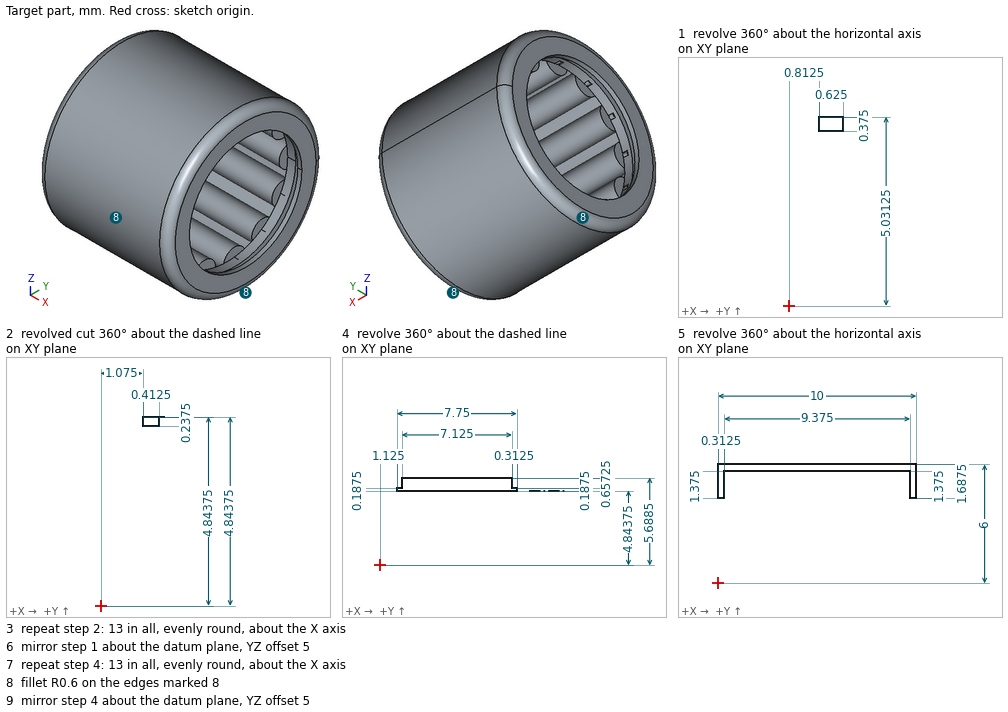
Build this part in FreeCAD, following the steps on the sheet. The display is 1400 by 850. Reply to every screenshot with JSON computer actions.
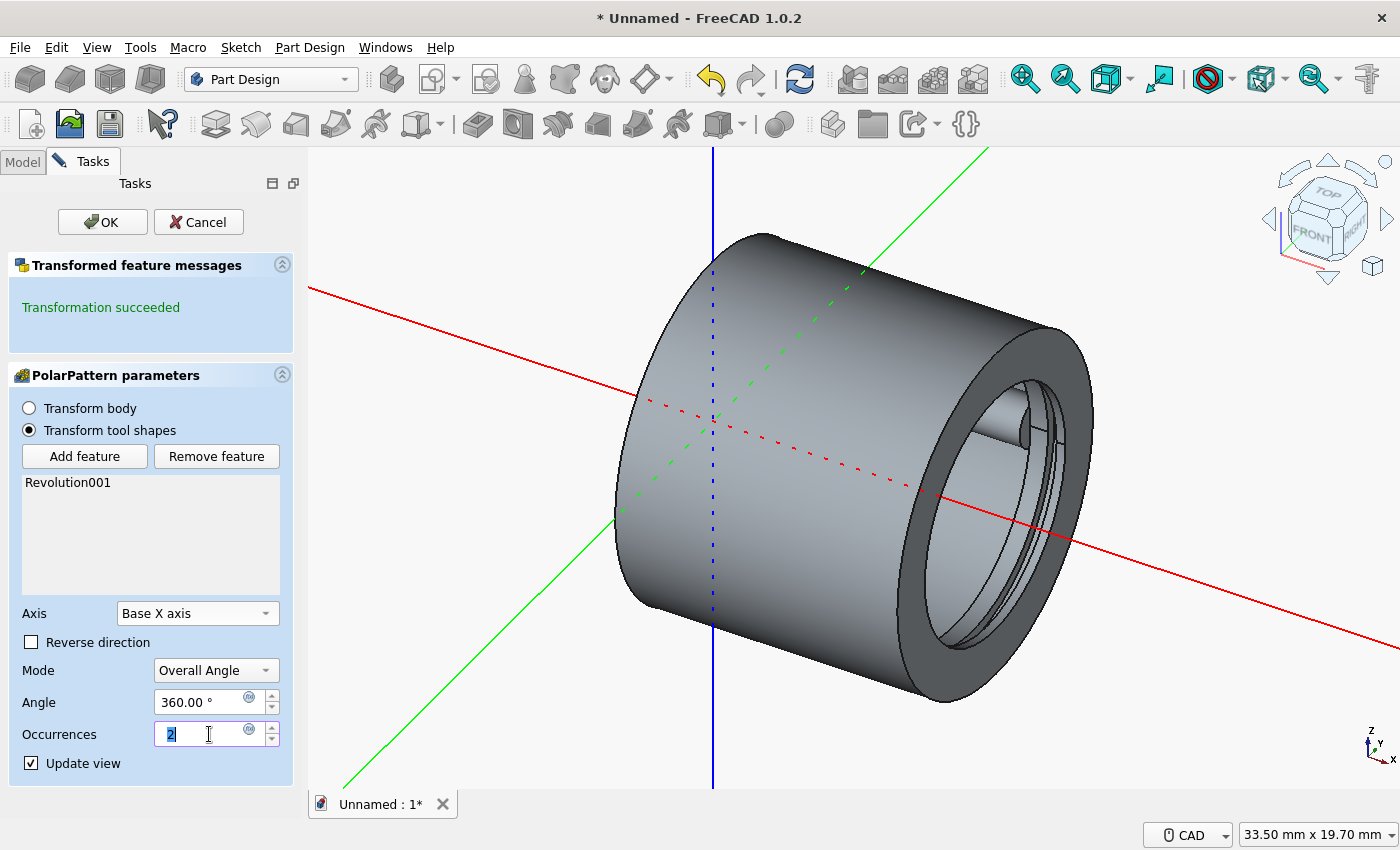
{"action": "type", "text": "13"}
{"action": "key", "text": "Tab"}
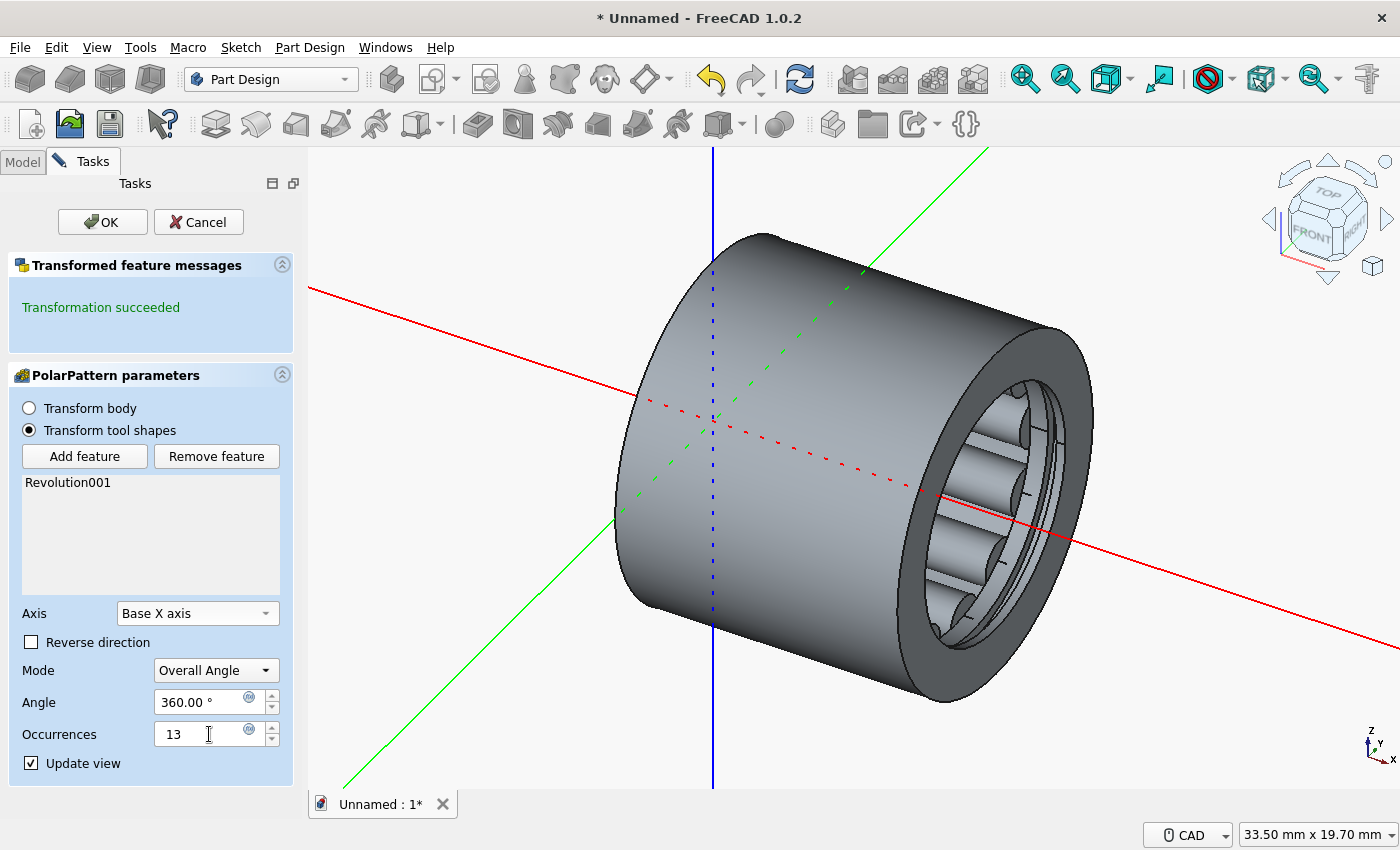
{"action": "left_click", "coordinate": [103, 222]}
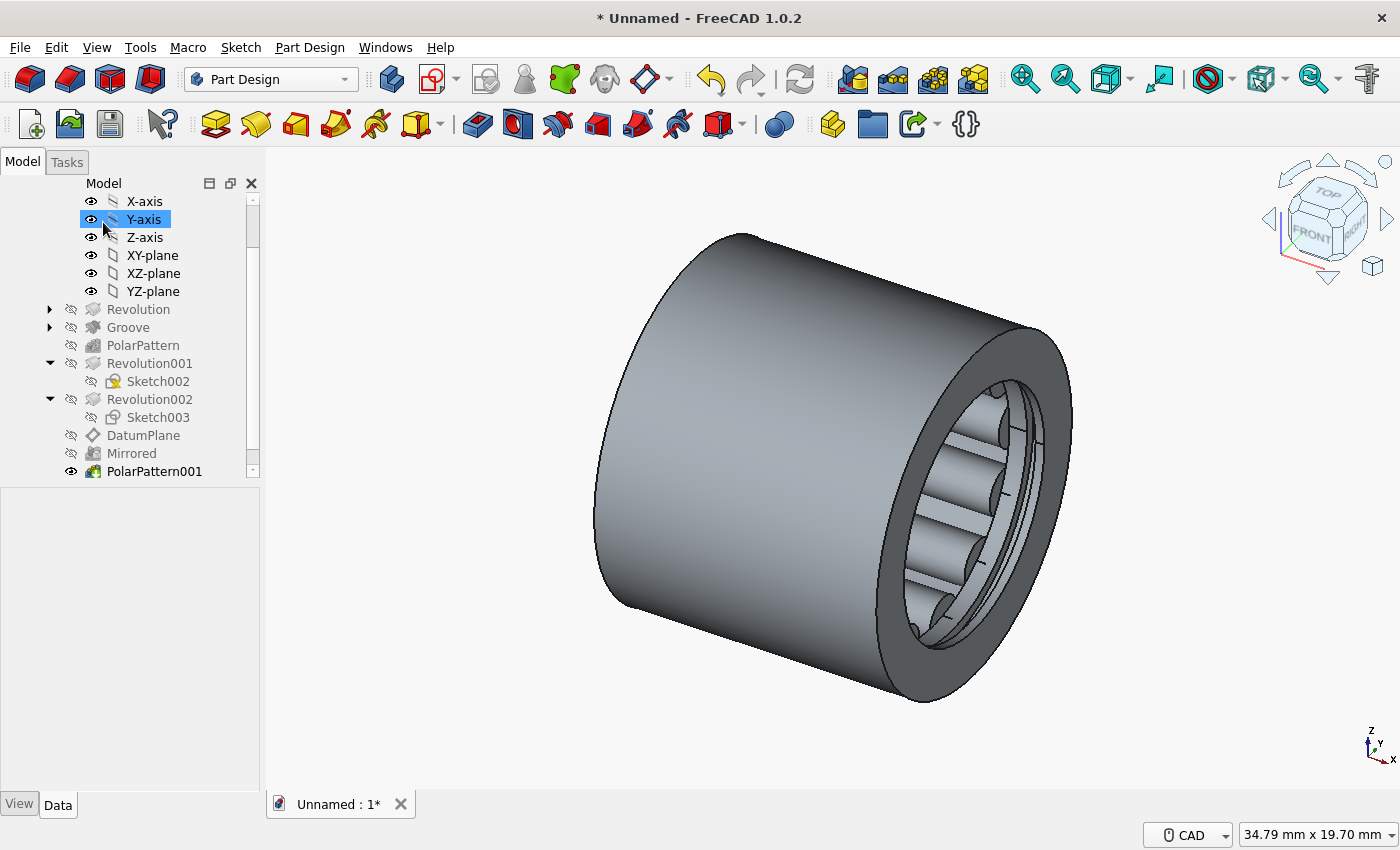
{"action": "left_click", "coordinate": [876, 611]}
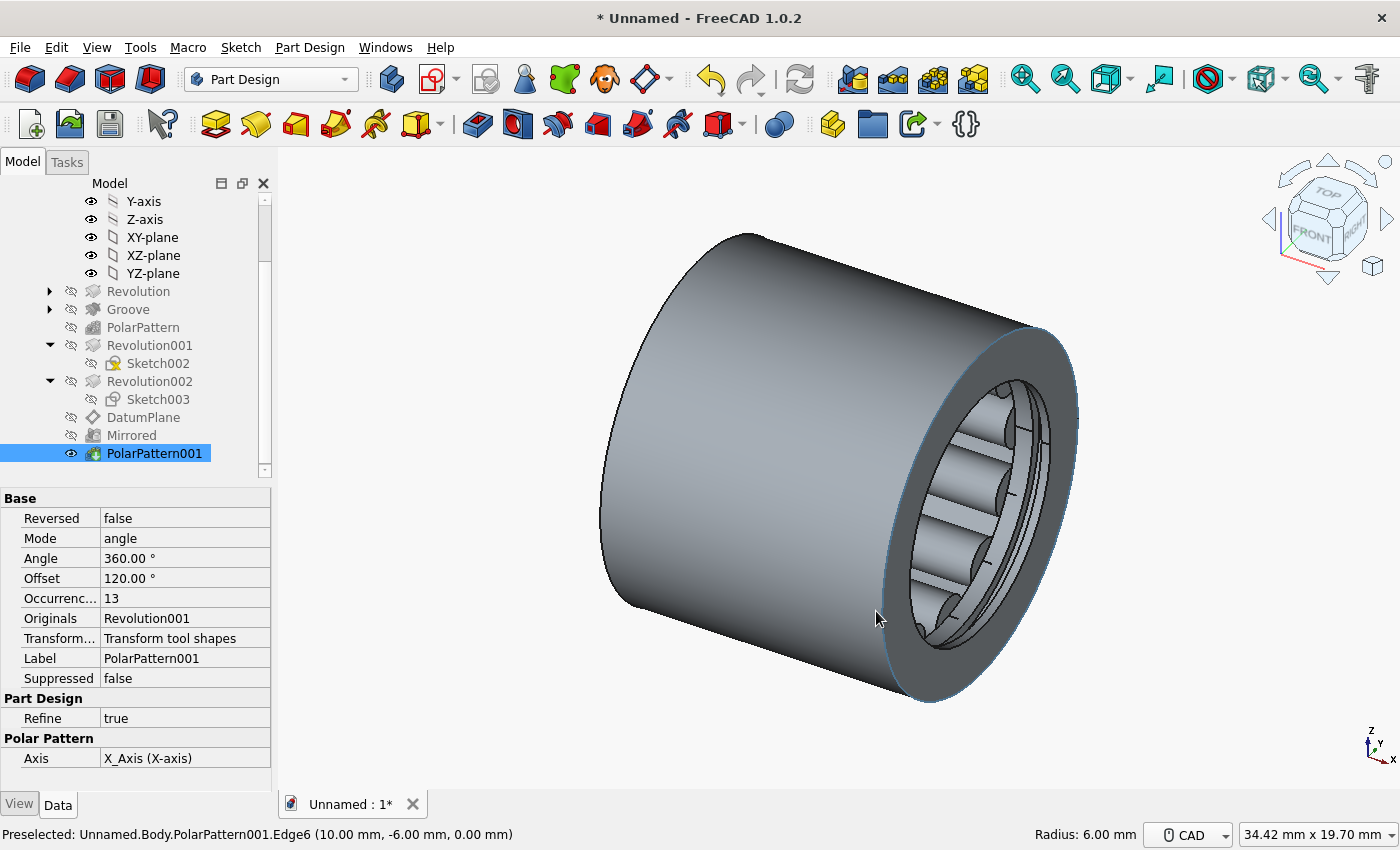
{"action": "key", "text": "0"}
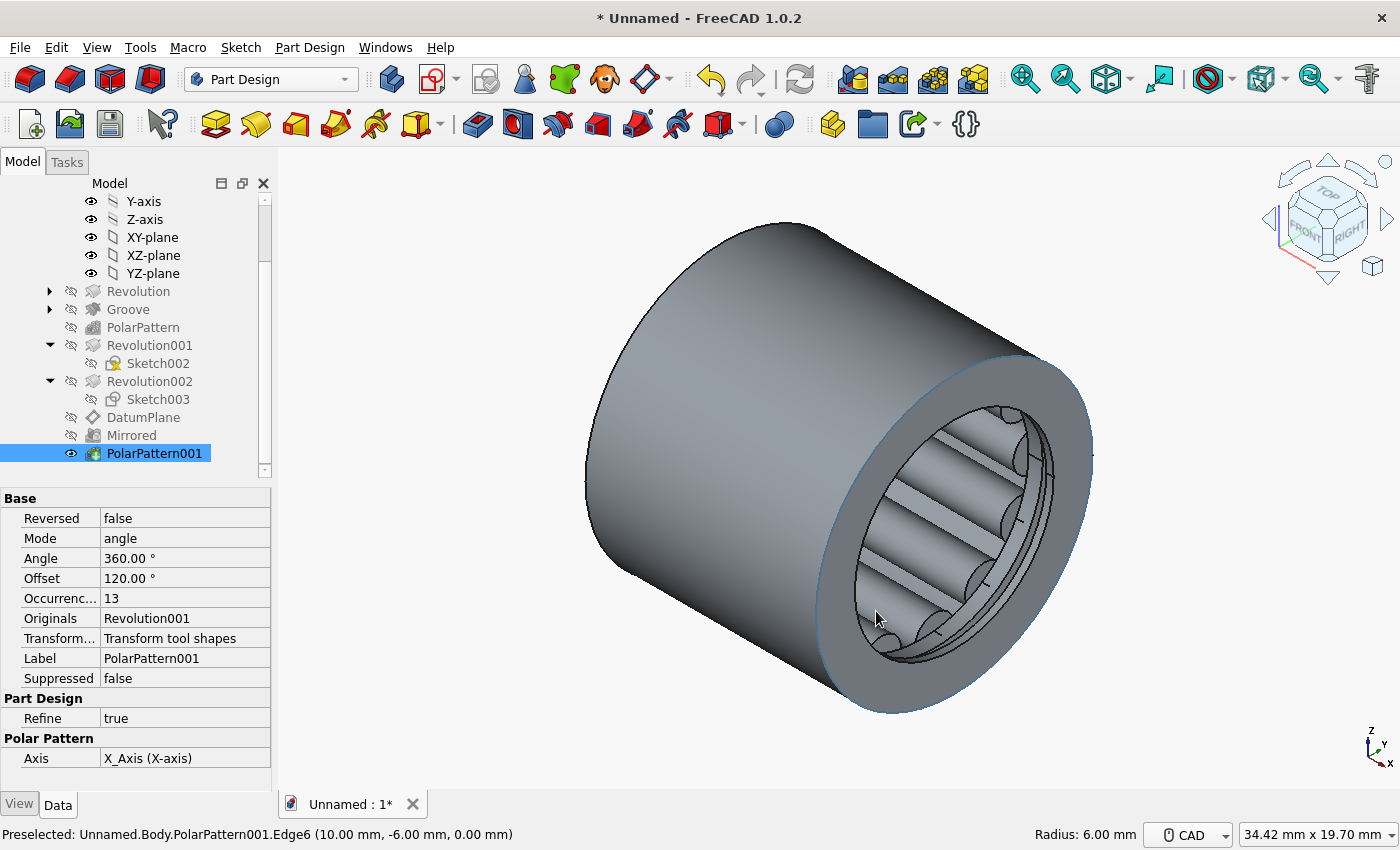
{"action": "key", "text": "2"}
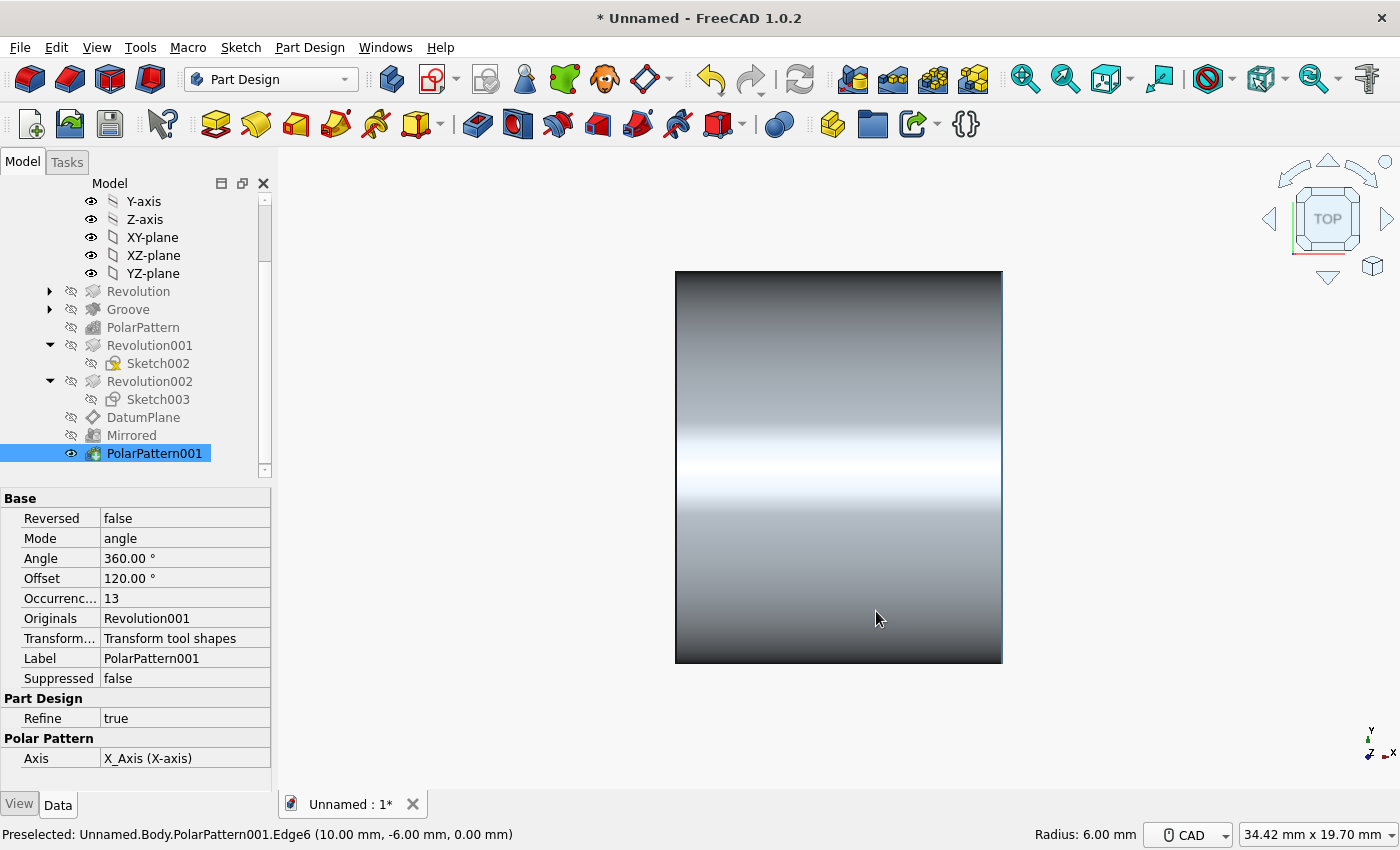
{"action": "left_click", "coordinate": [676, 625], "text": "ctrl"}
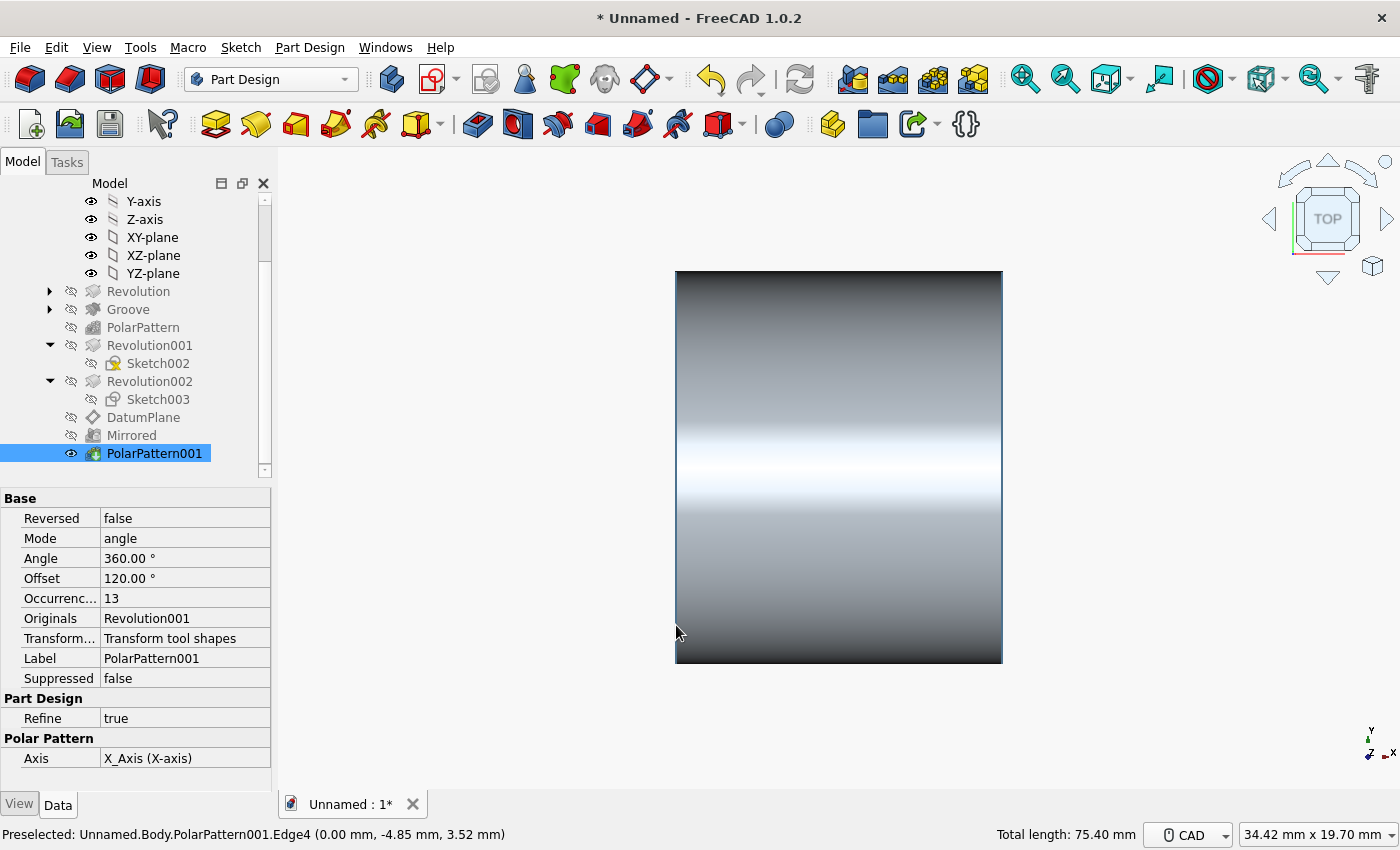
{"action": "left_click", "coordinate": [30, 80]}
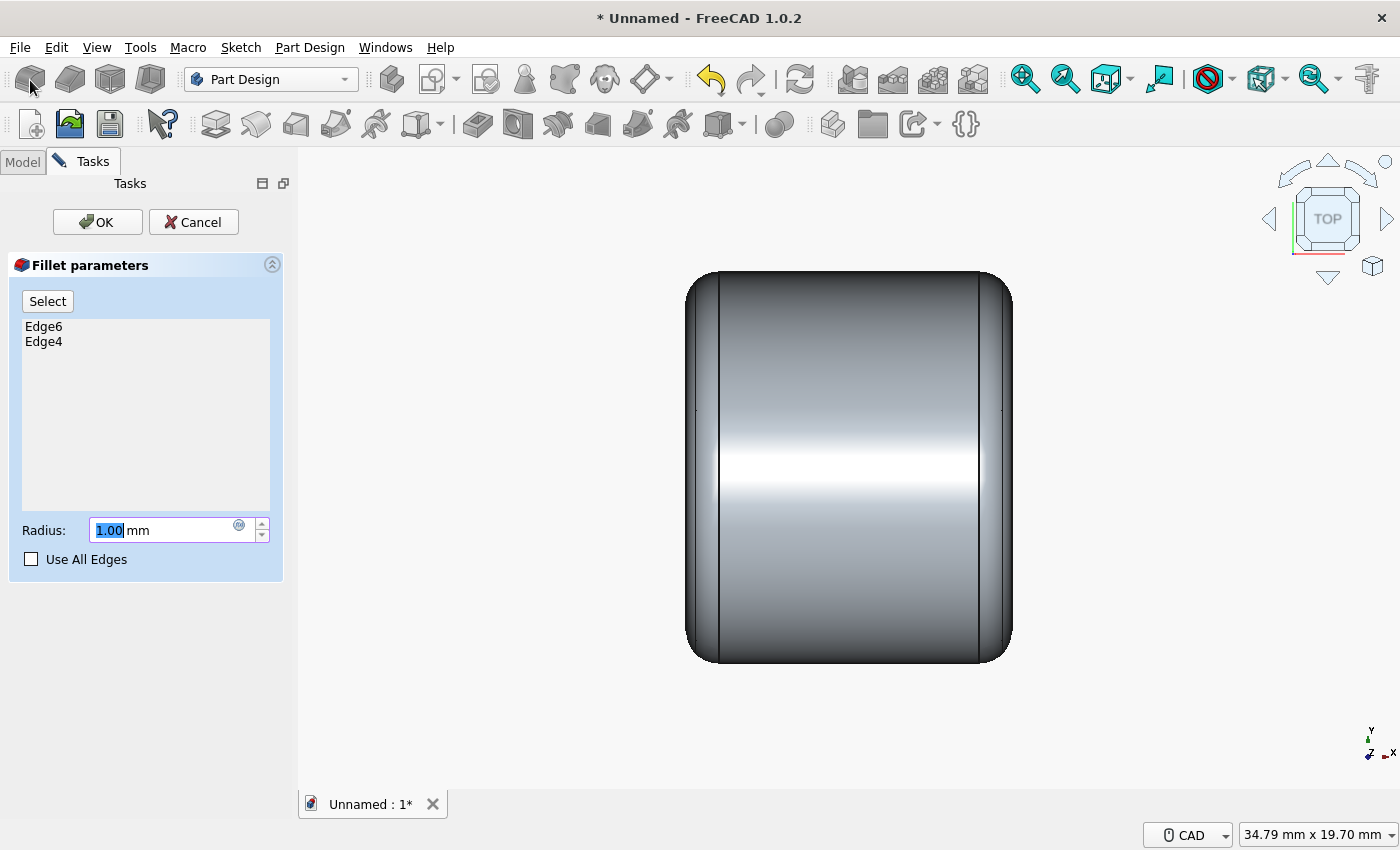
{"action": "type", "text": "0.6"}
{"action": "key", "text": "Tab"}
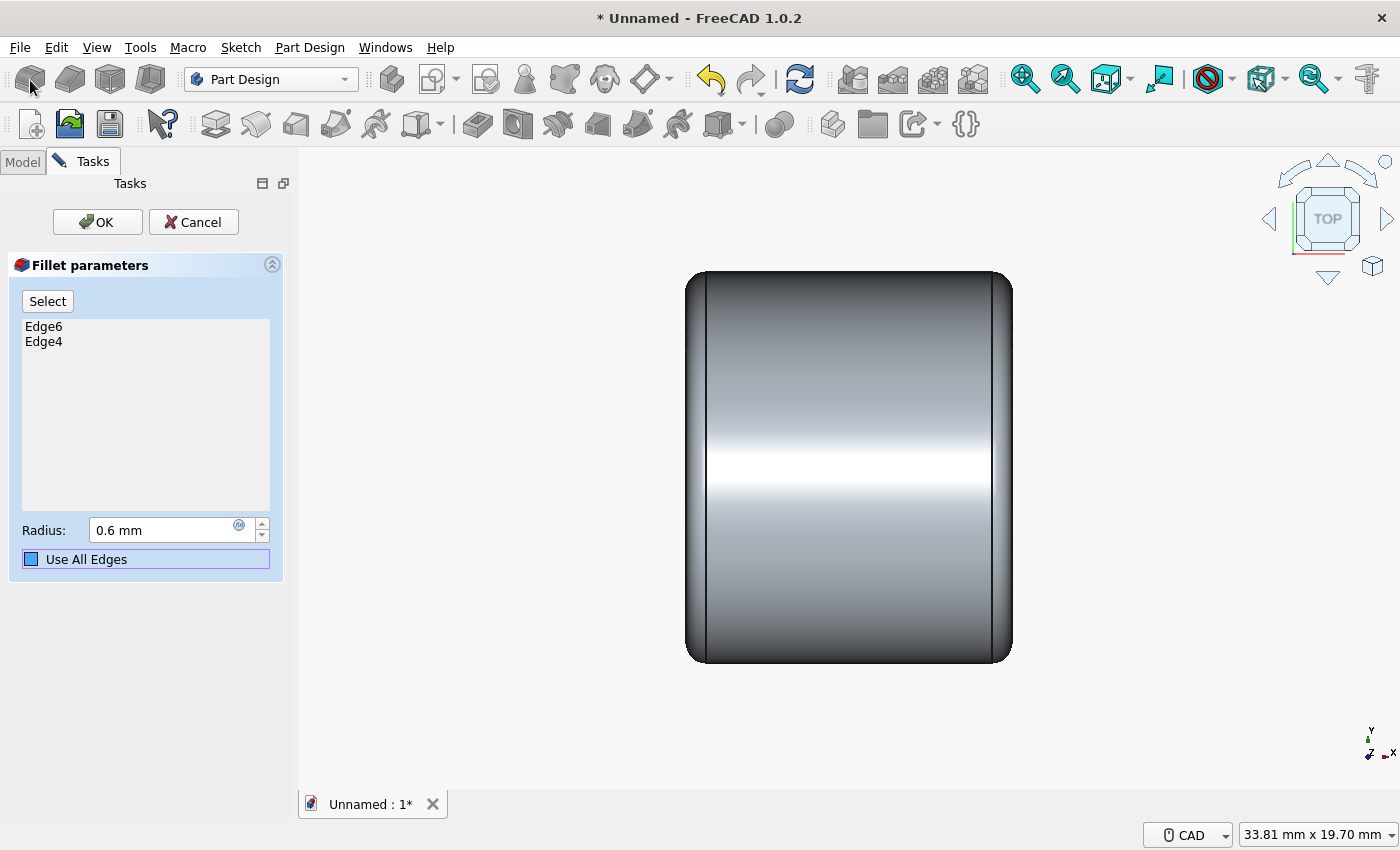
{"action": "left_click", "coordinate": [98, 222]}